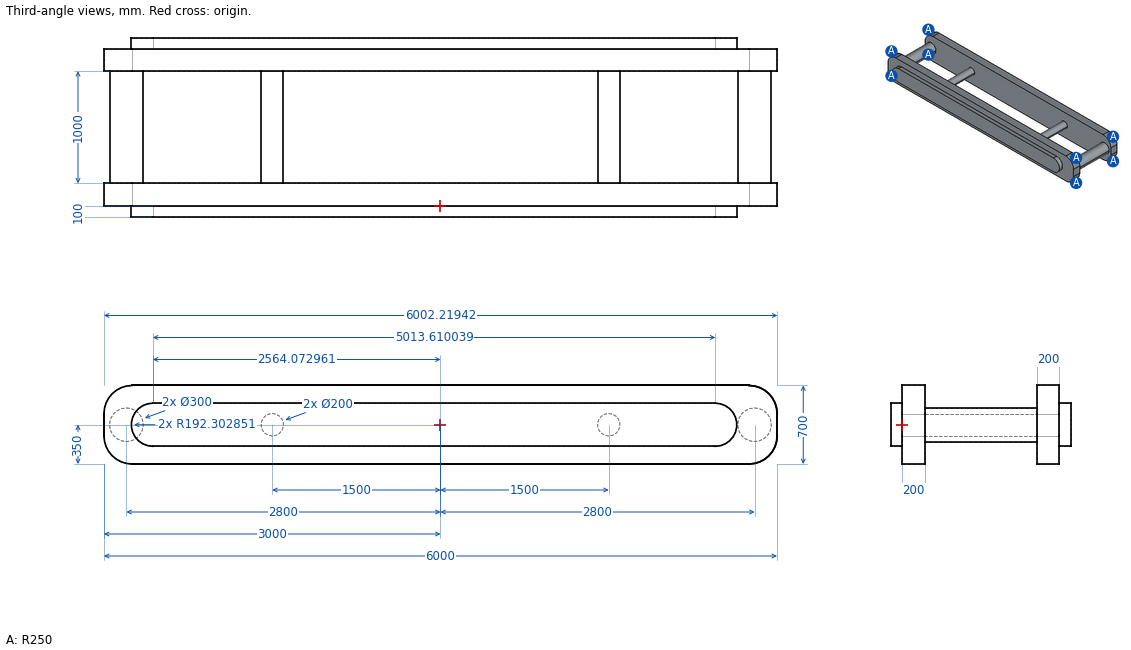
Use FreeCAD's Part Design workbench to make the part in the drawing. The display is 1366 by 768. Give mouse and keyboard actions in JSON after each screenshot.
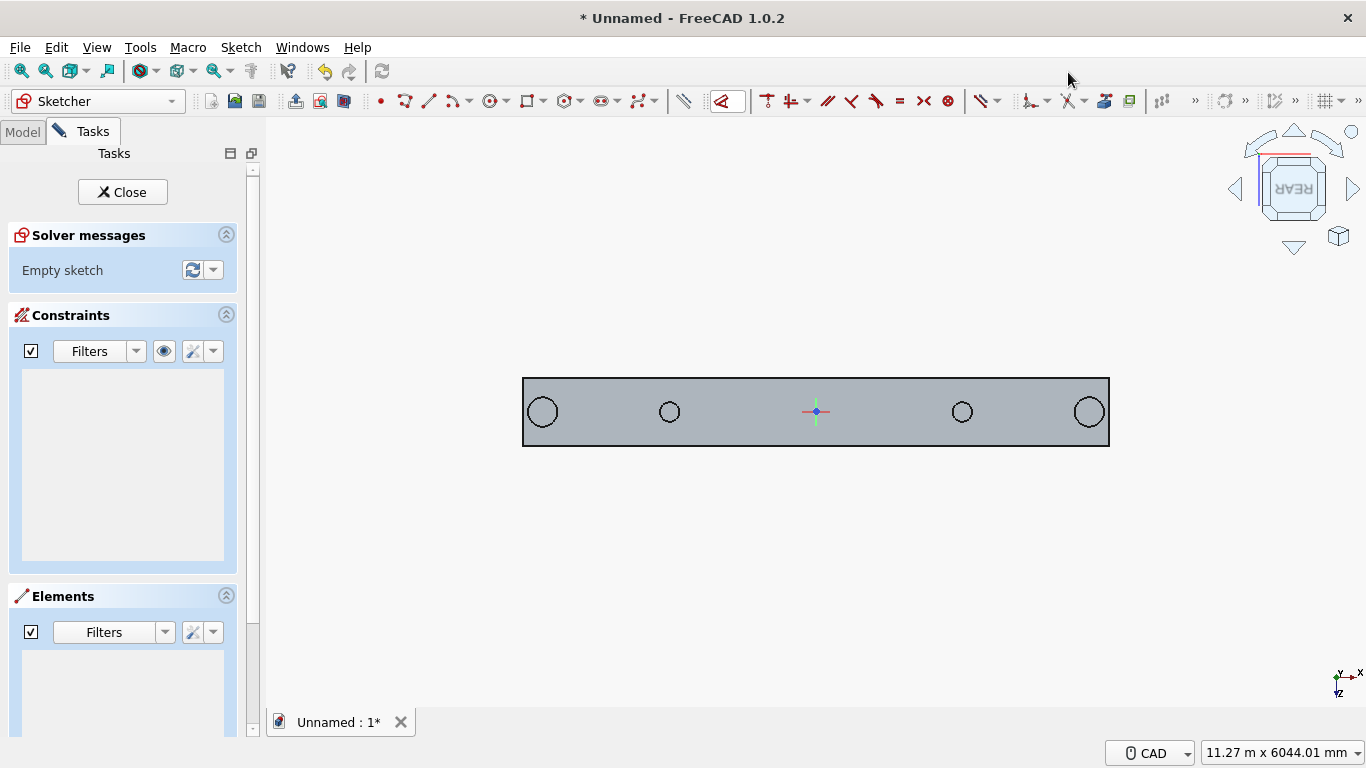
{"action": "left_click", "coordinate": [528, 102]}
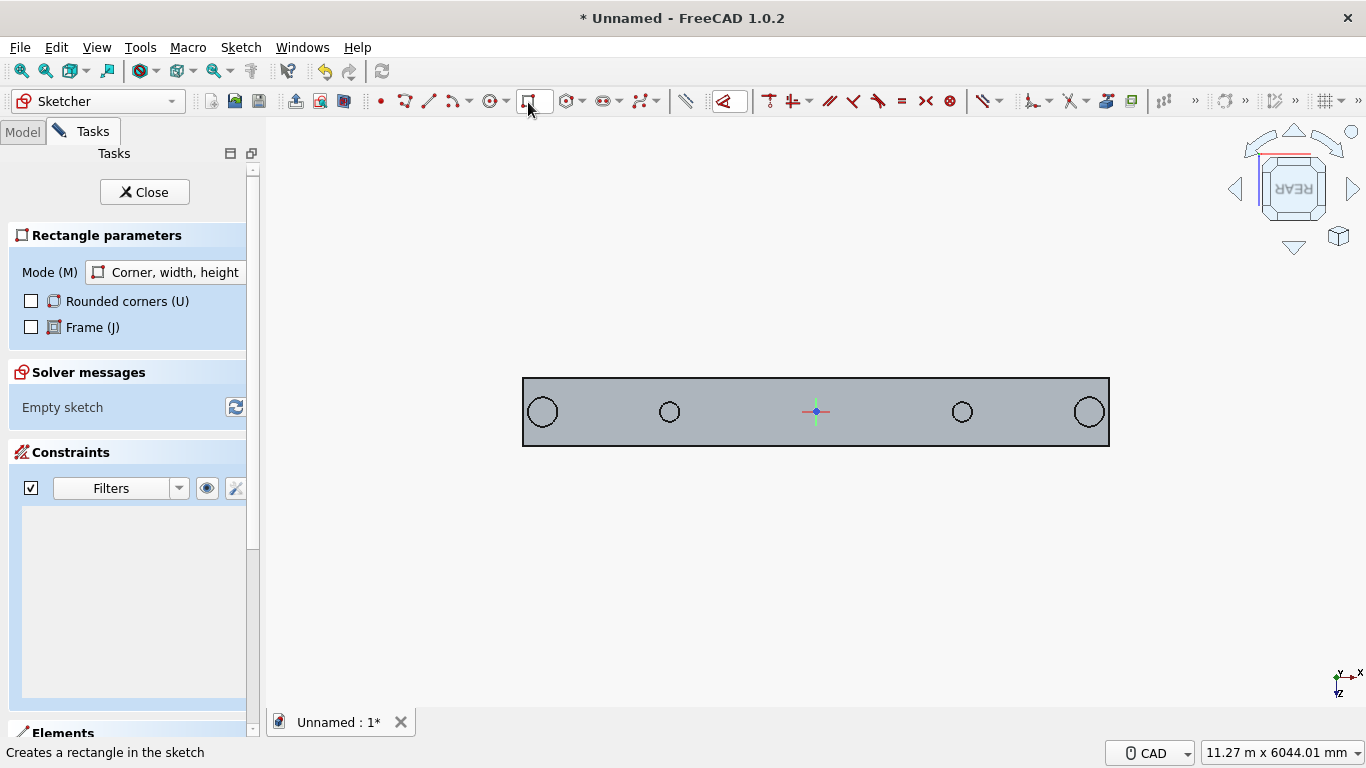
{"action": "left_click", "coordinate": [523, 378]}
{"action": "left_click", "coordinate": [1109, 446]}
{"action": "key", "text": "Escape"}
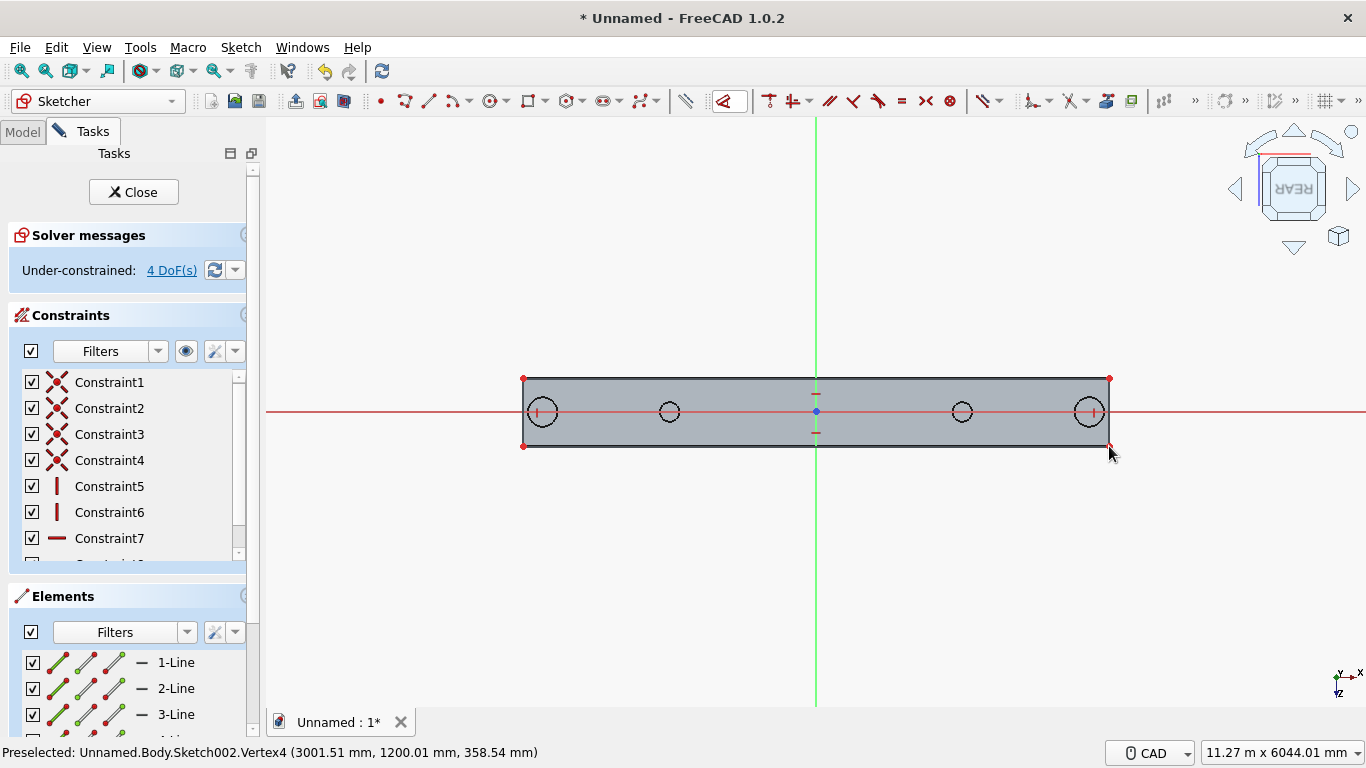
{"action": "left_click", "coordinate": [523, 399]}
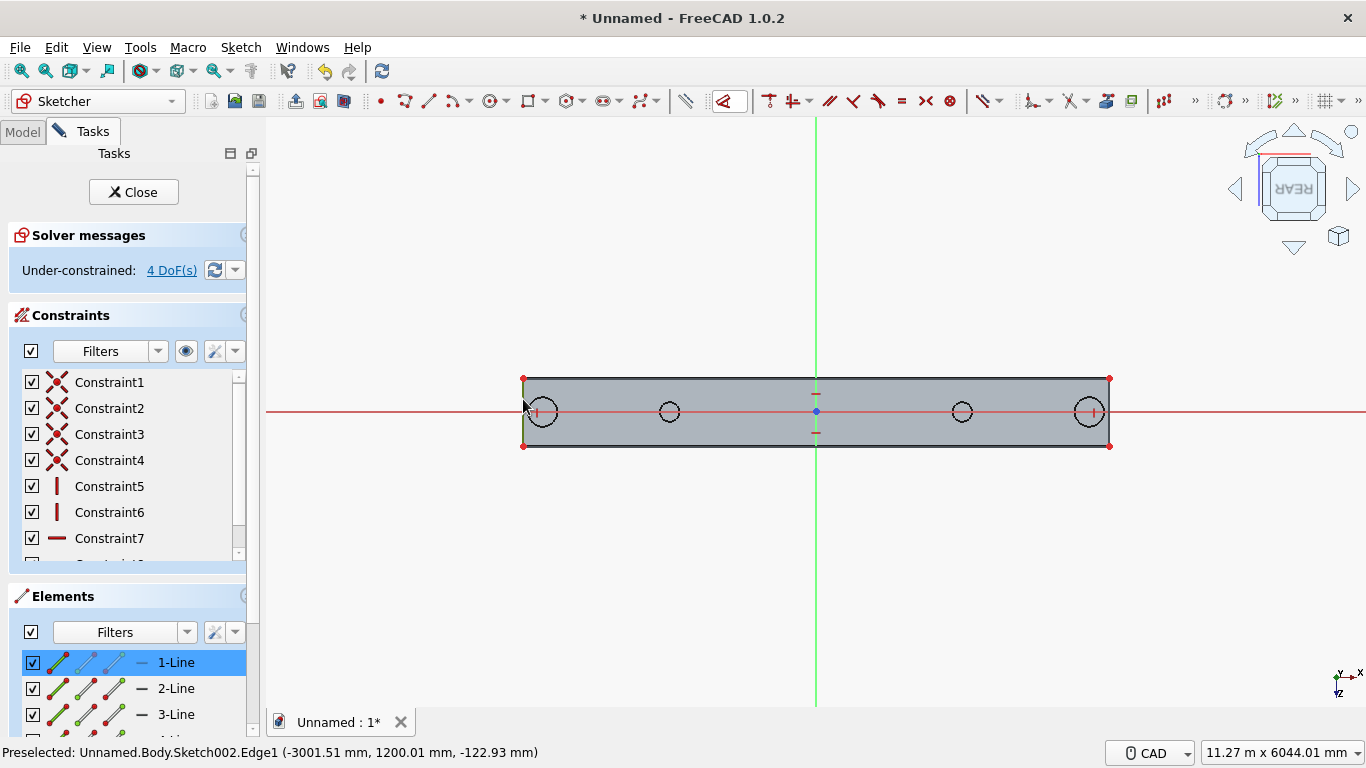
{"action": "key", "text": "i"}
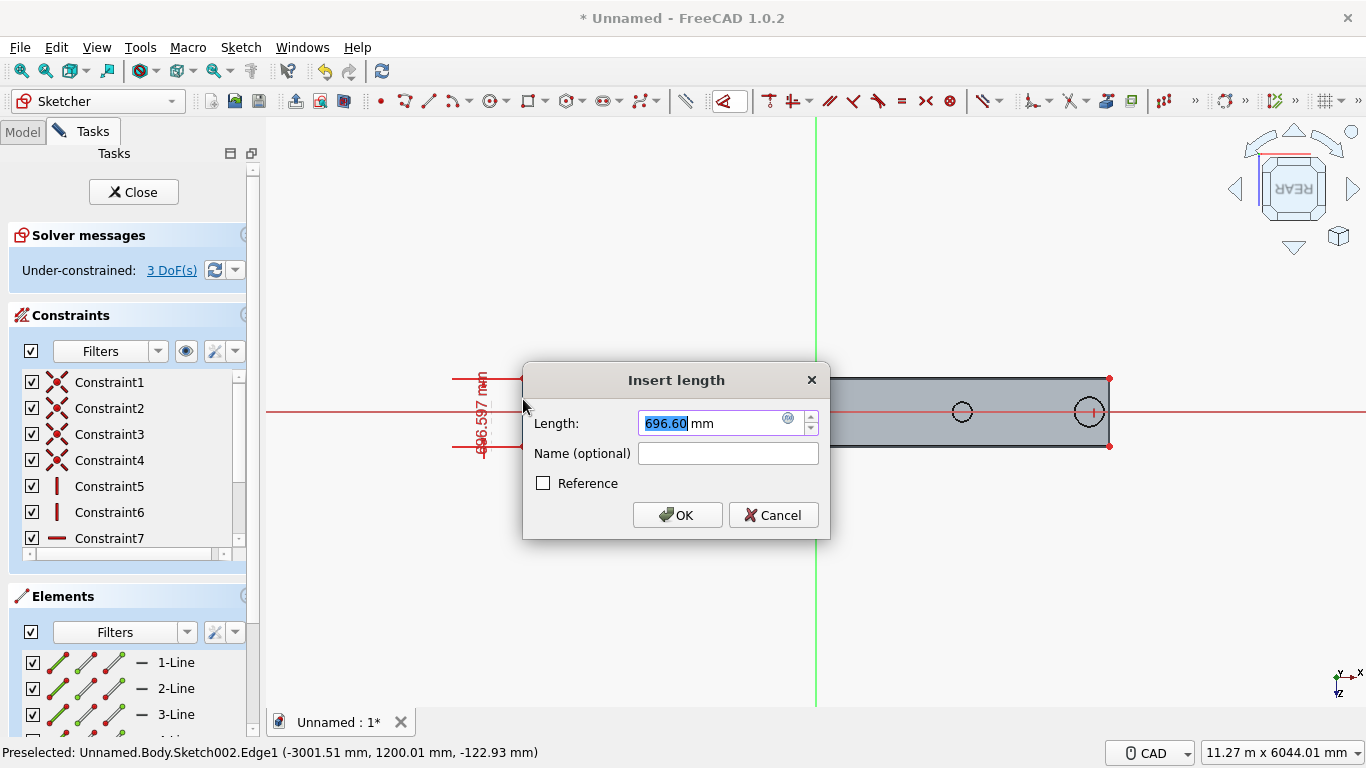
{"action": "type", "text": "700"}
{"action": "key", "text": "Return"}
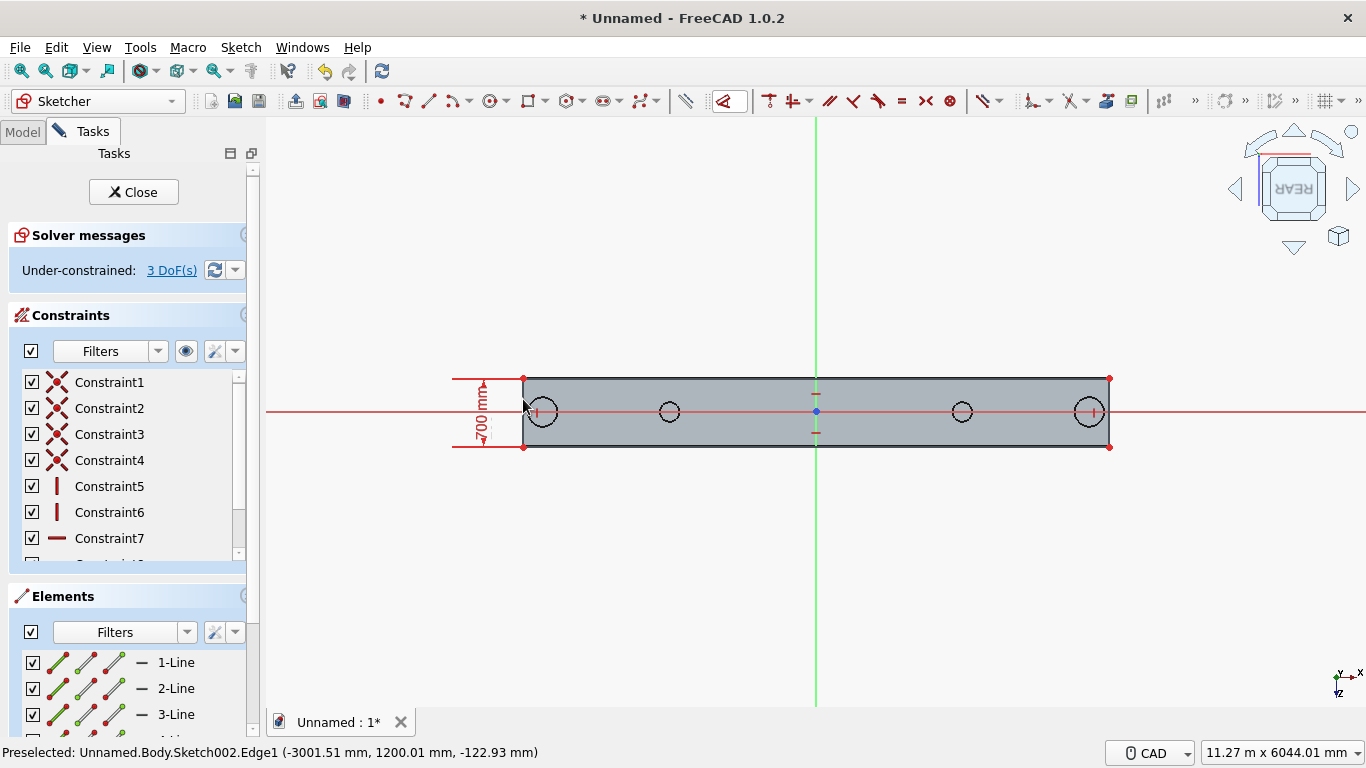
{"action": "left_click", "coordinate": [523, 379]}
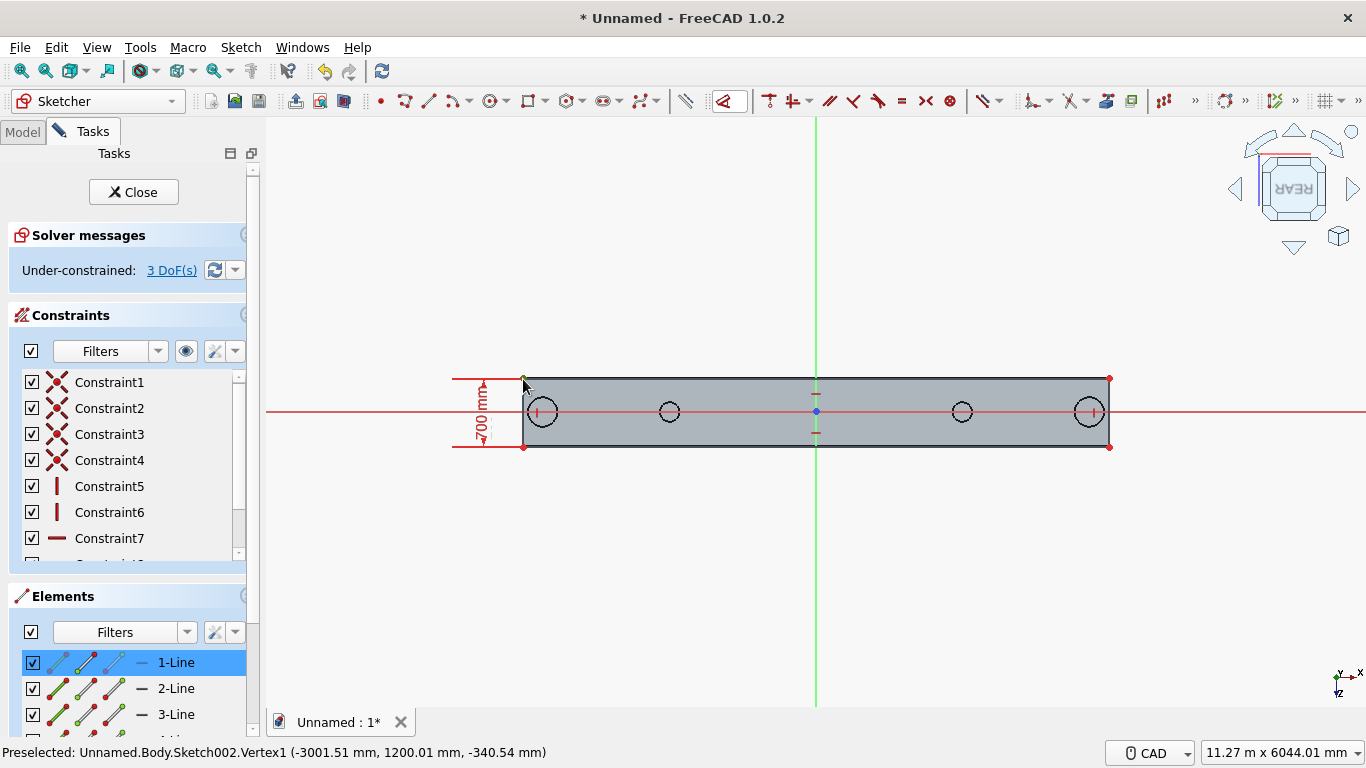
{"action": "left_click", "coordinate": [742, 102]}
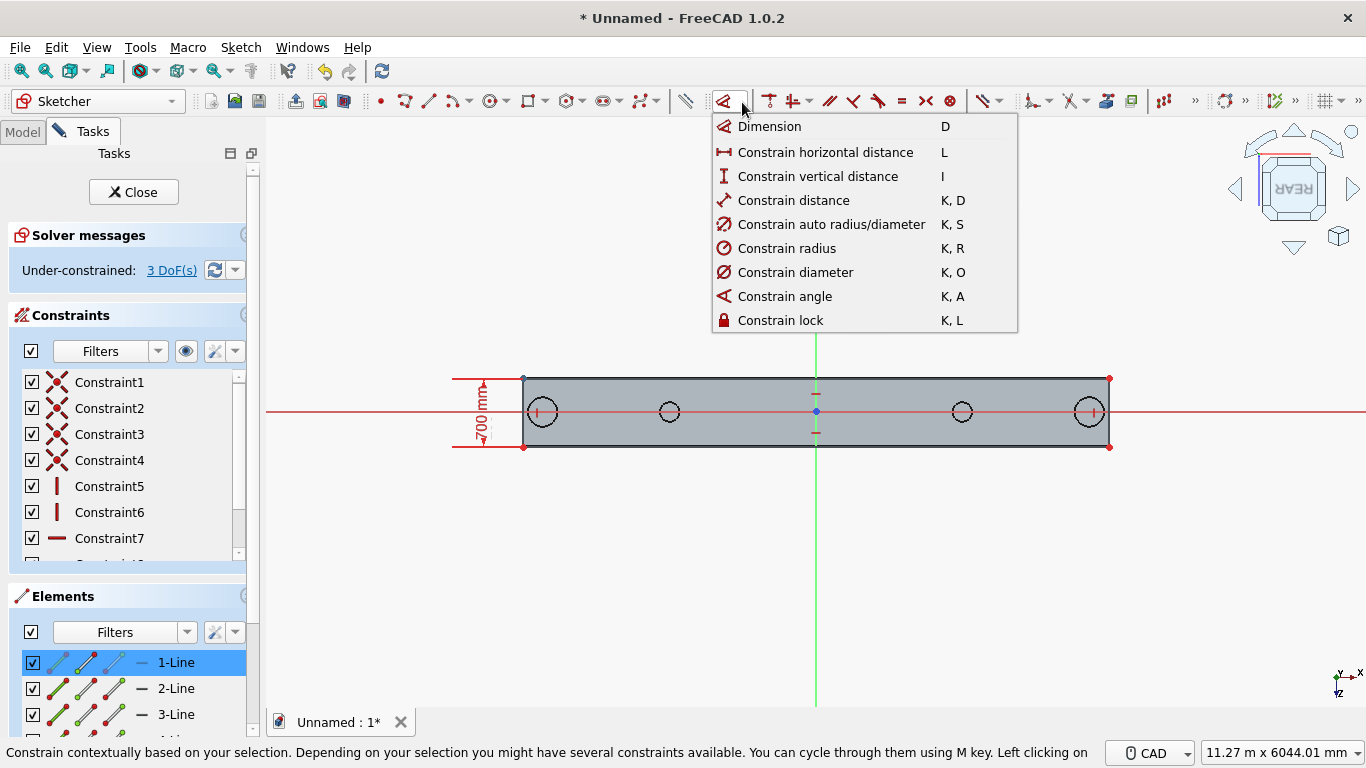
{"action": "left_click", "coordinate": [865, 176]}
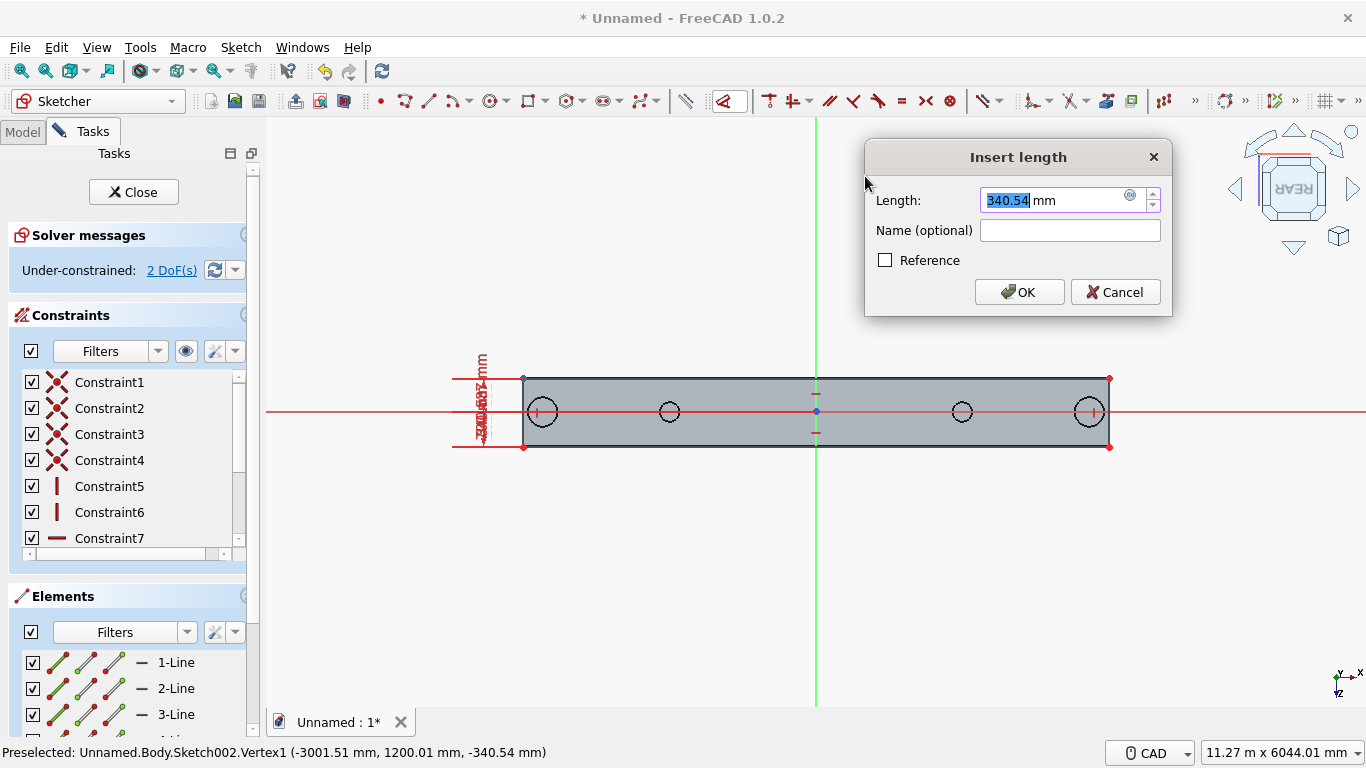
{"action": "type", "text": "350"}
{"action": "key", "text": "Return"}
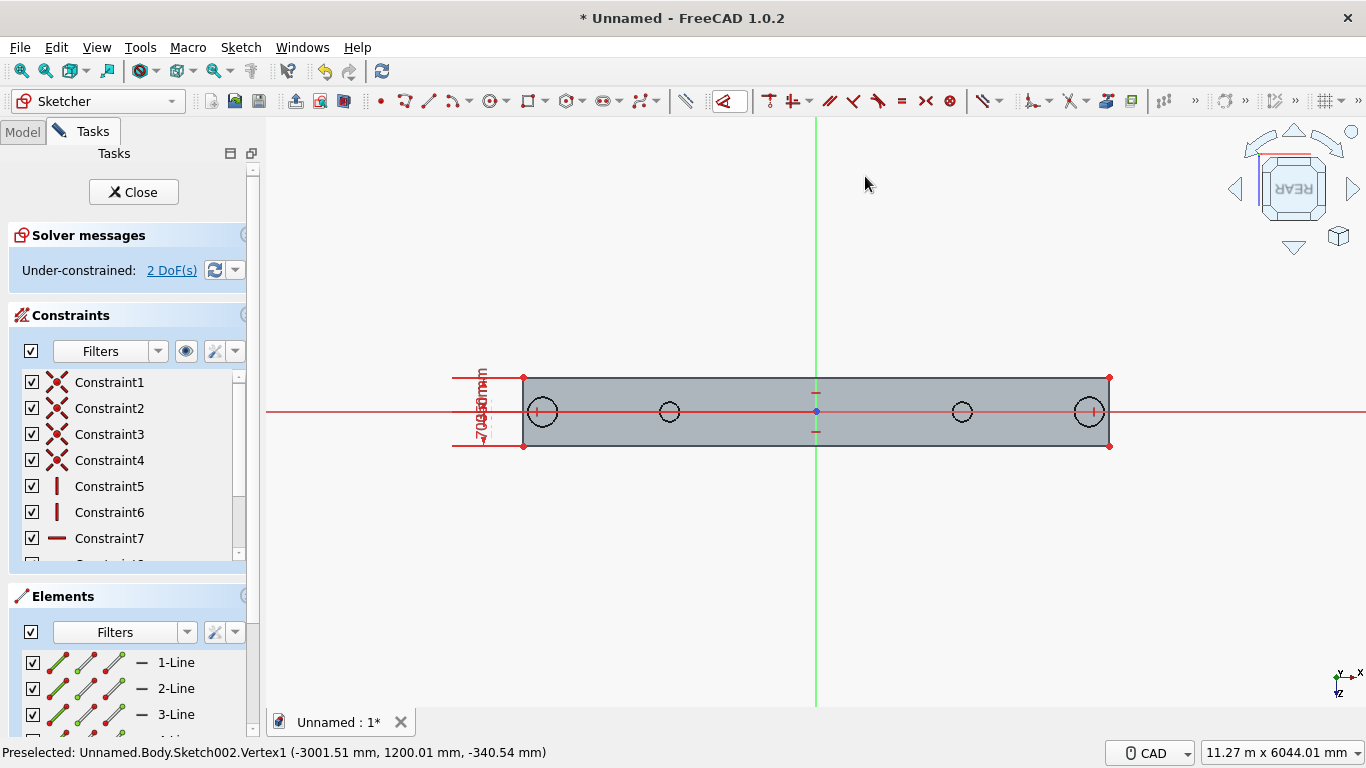
{"action": "left_click", "coordinate": [523, 378]}